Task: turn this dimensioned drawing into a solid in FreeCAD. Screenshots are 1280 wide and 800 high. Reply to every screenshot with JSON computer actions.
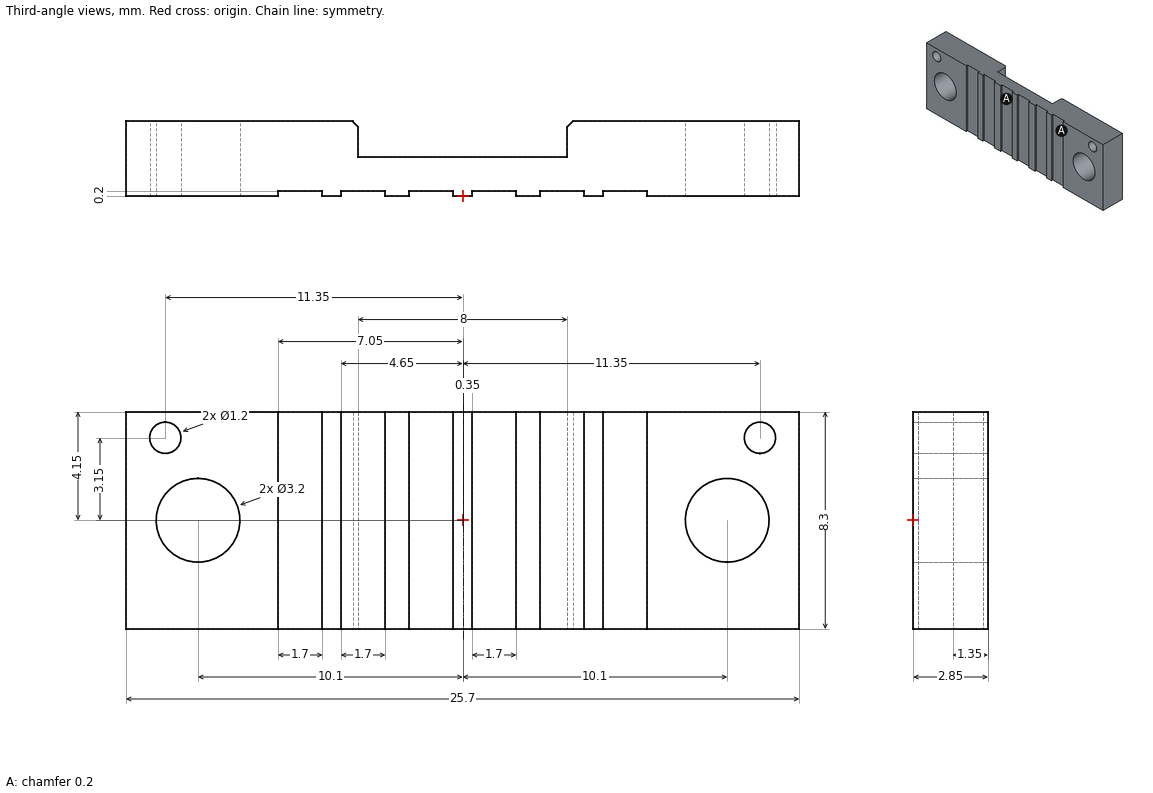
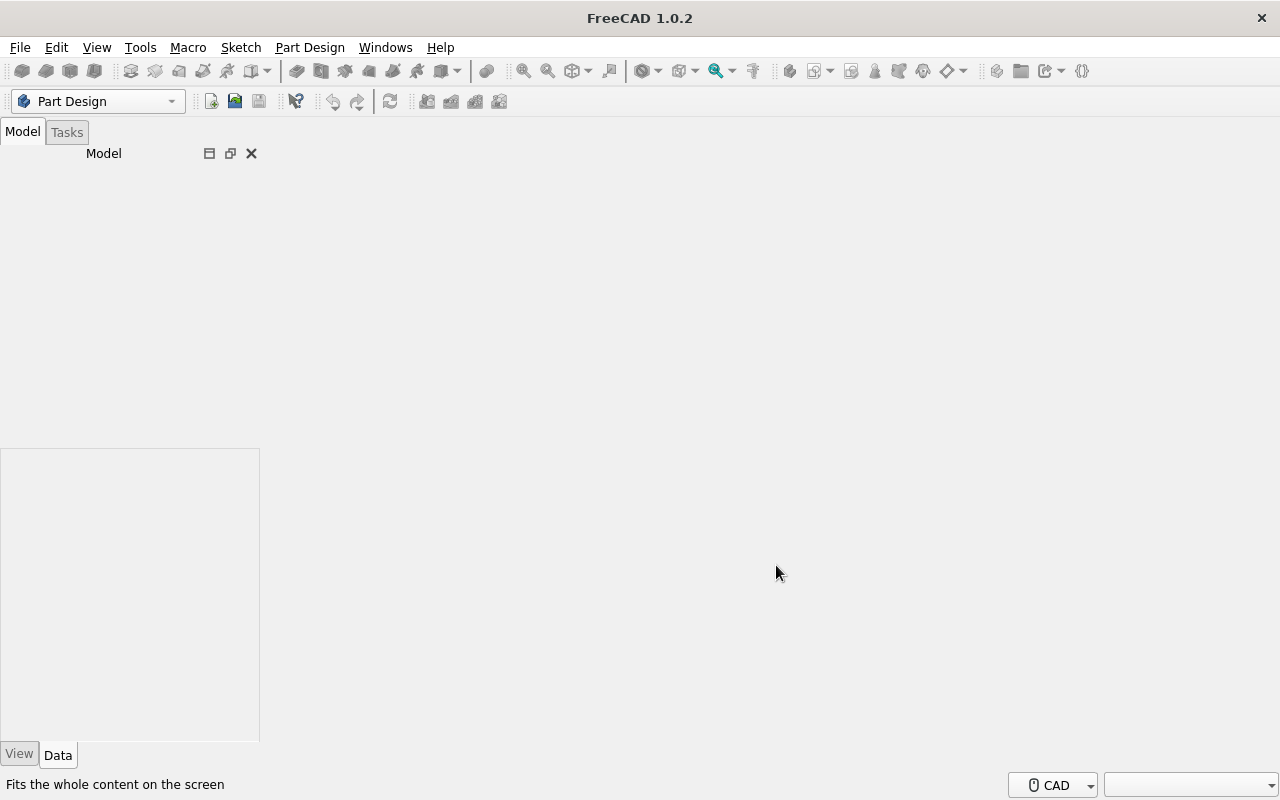
{"action": "left_click", "coordinate": [212, 102]}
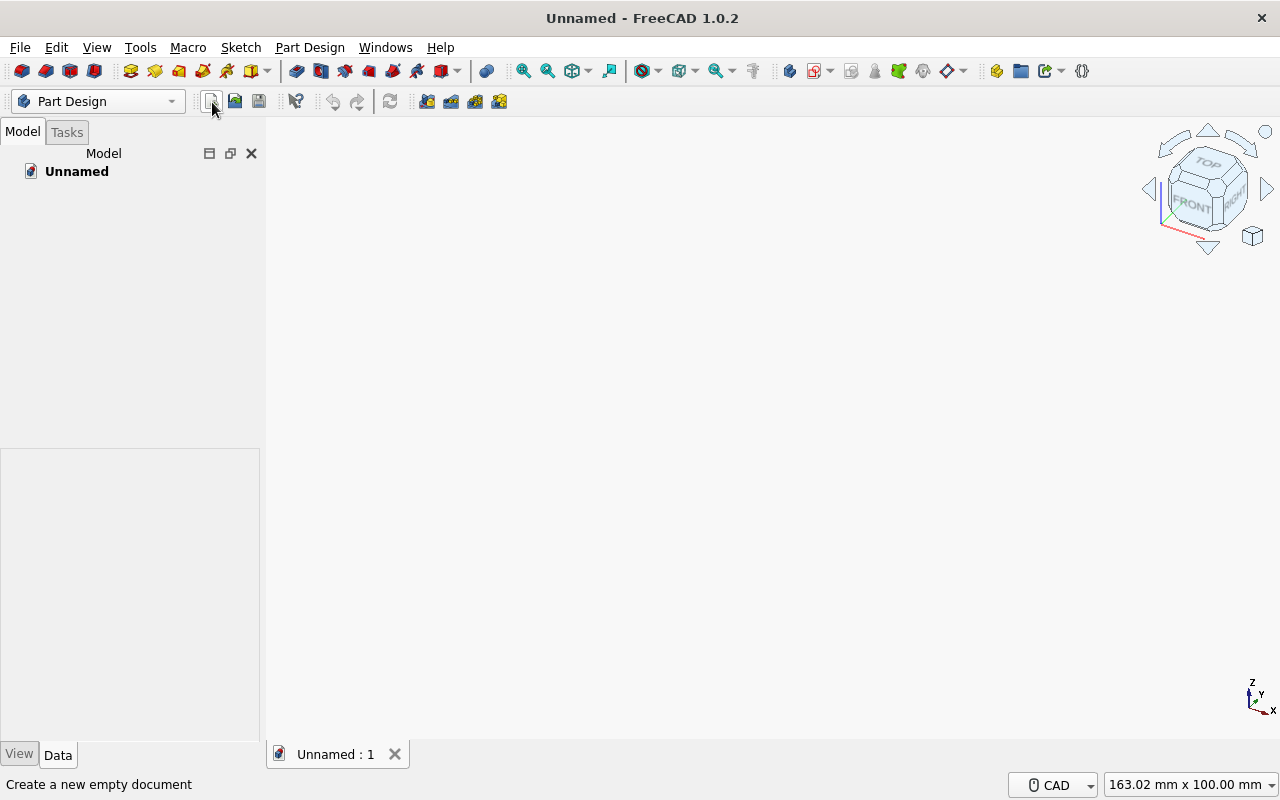
{"action": "left_click", "coordinate": [814, 72]}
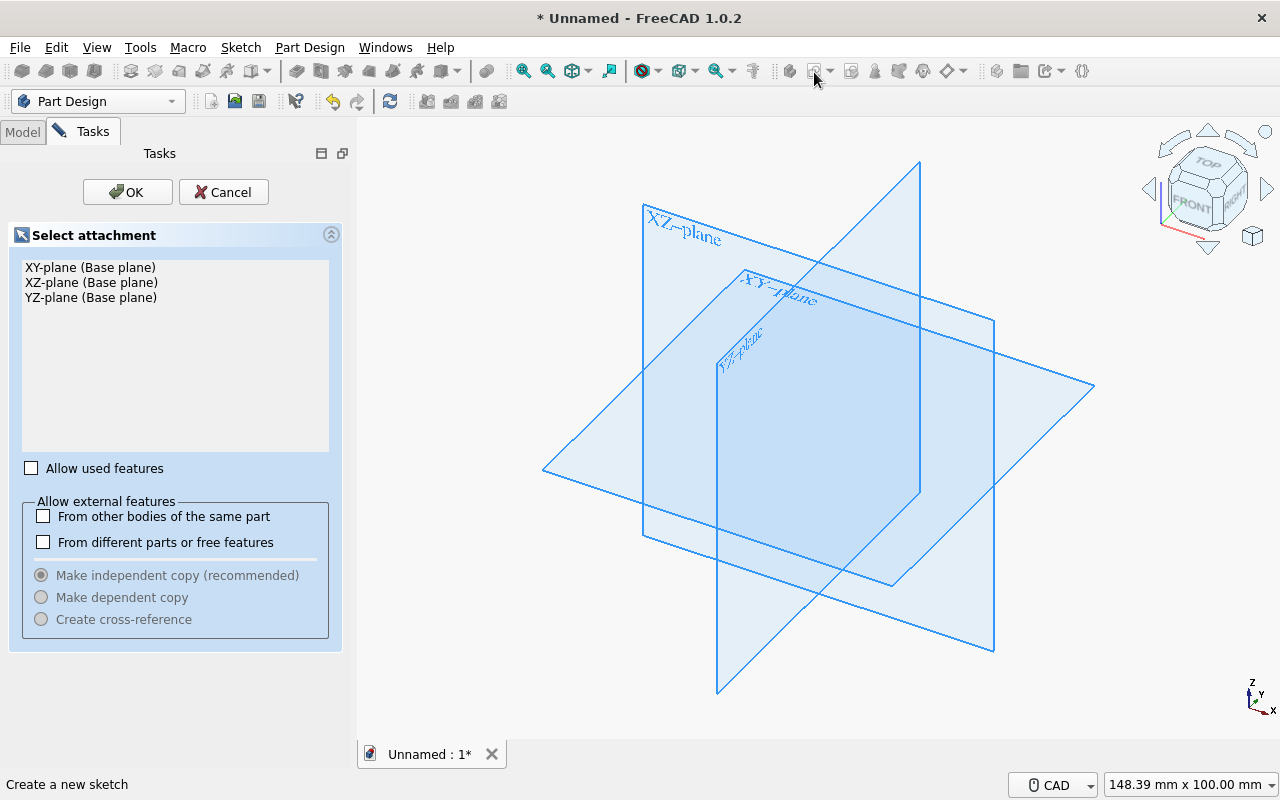
{"action": "left_click", "coordinate": [82, 282]}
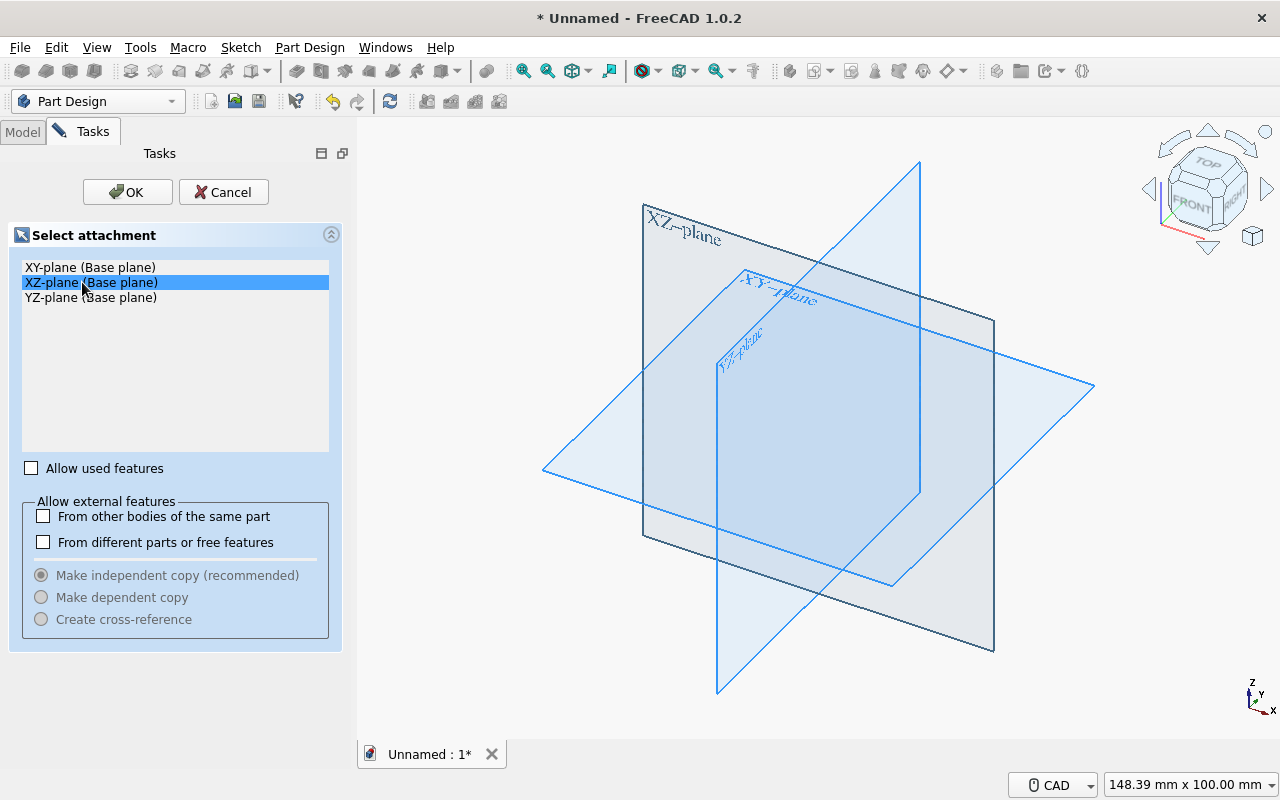
{"action": "left_click", "coordinate": [128, 192]}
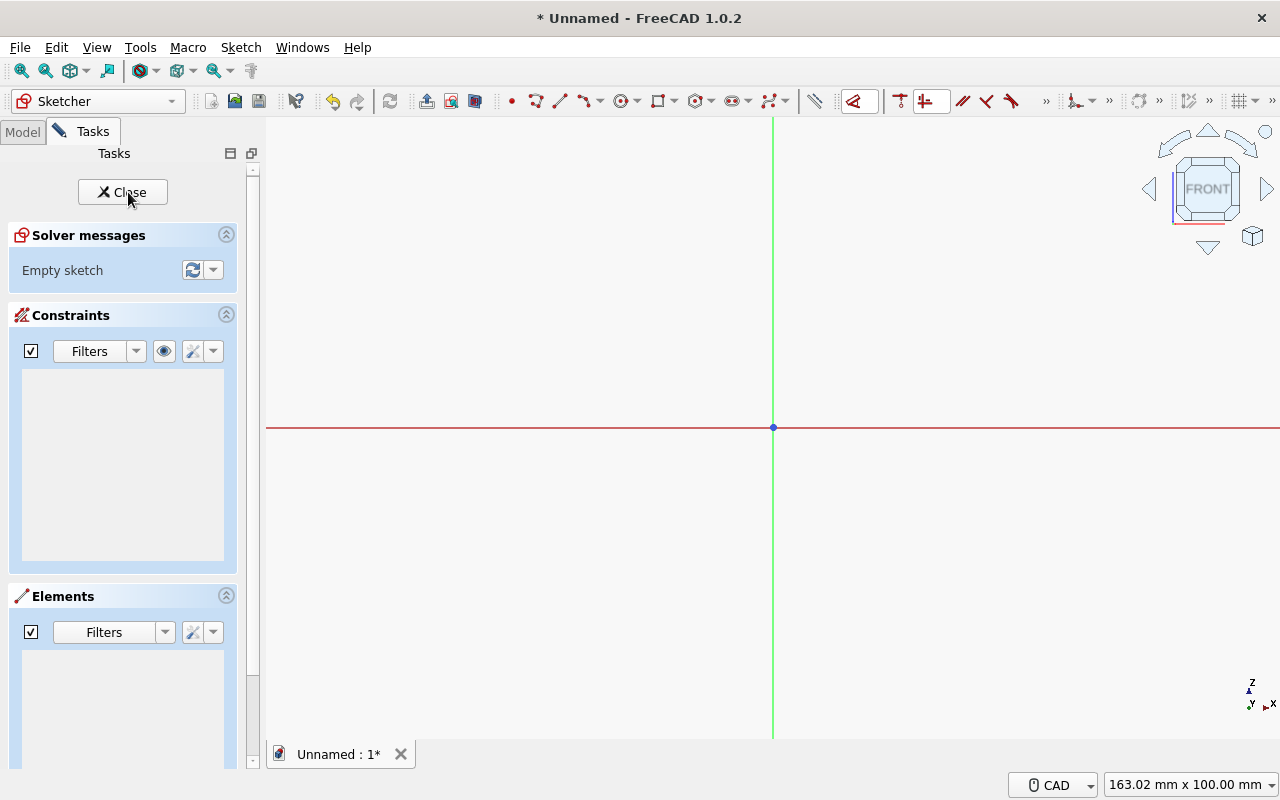
{"action": "scroll", "coordinate": [803, 428], "scroll_direction": "up", "scroll_amount": 6}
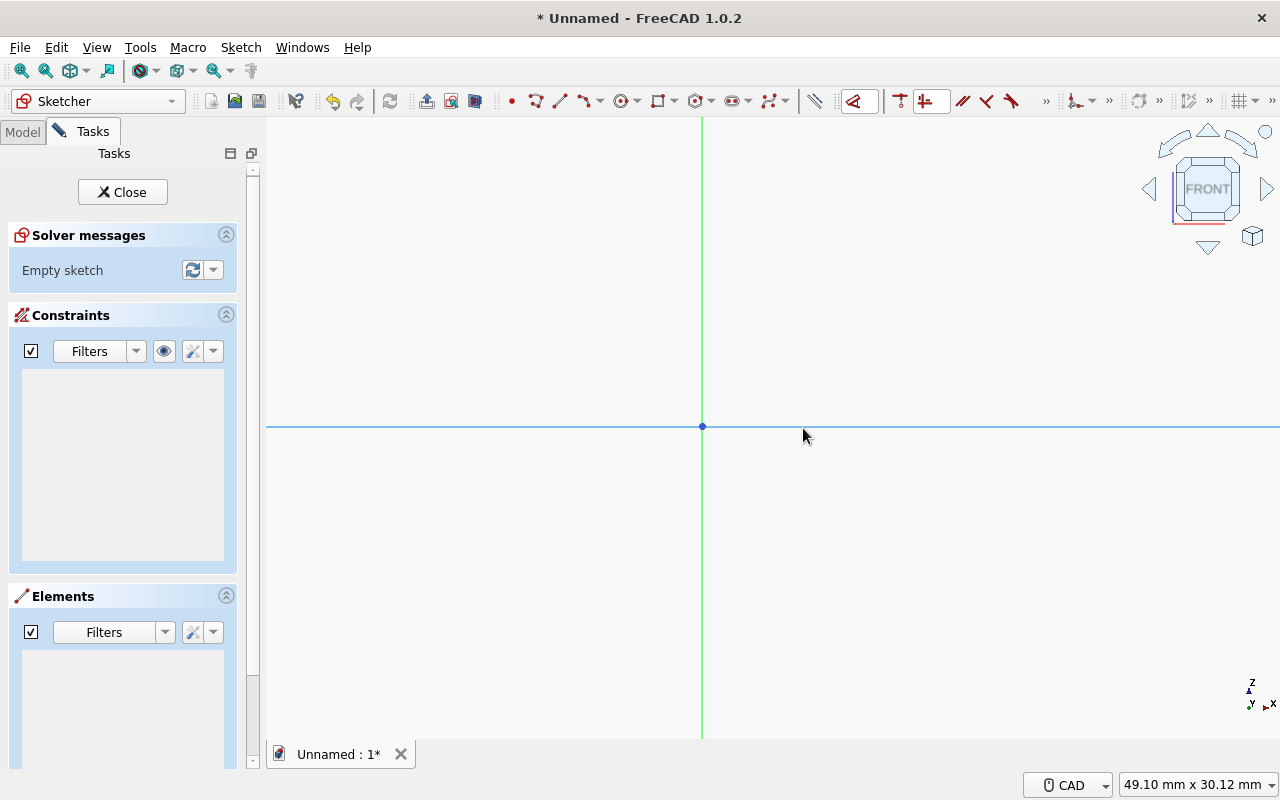
{"action": "key", "text": "g v"}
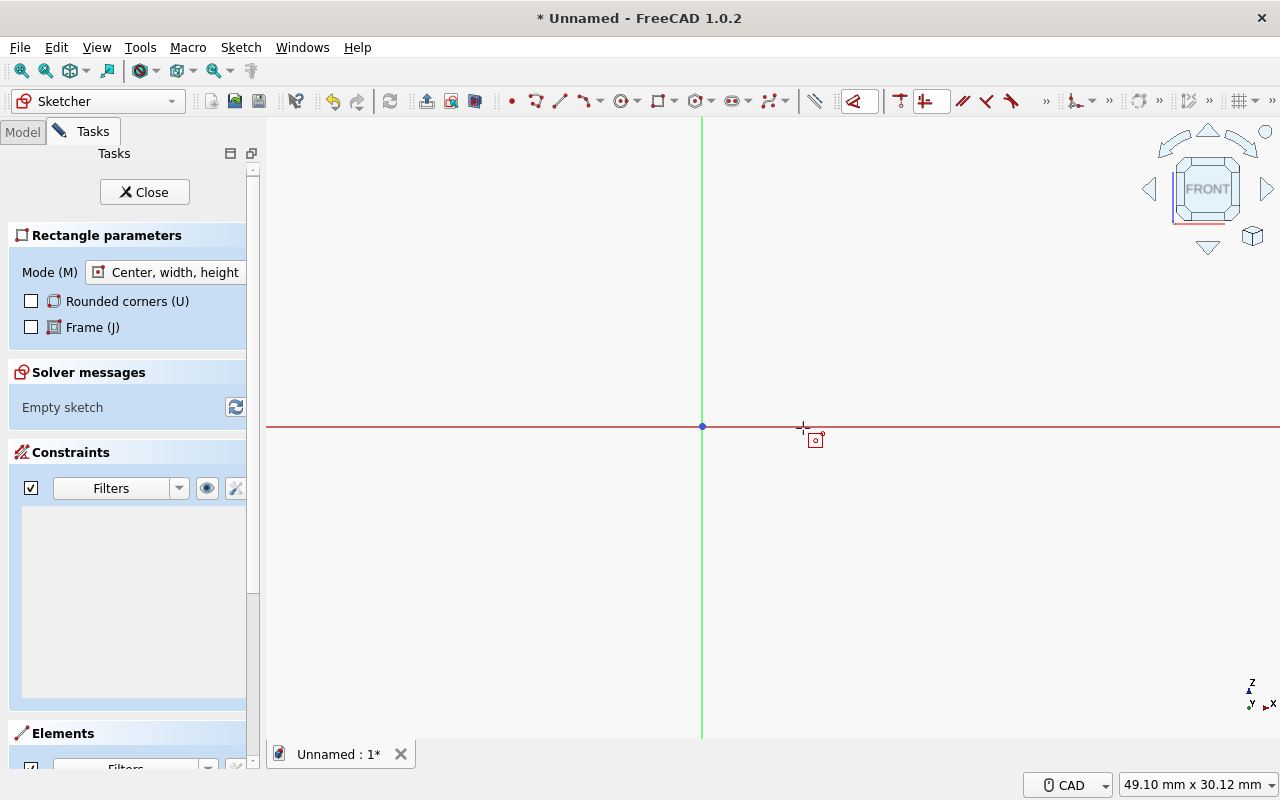
{"action": "left_click", "coordinate": [702, 427]}
{"action": "left_click", "coordinate": [968, 341]}
{"action": "key", "text": "Escape"}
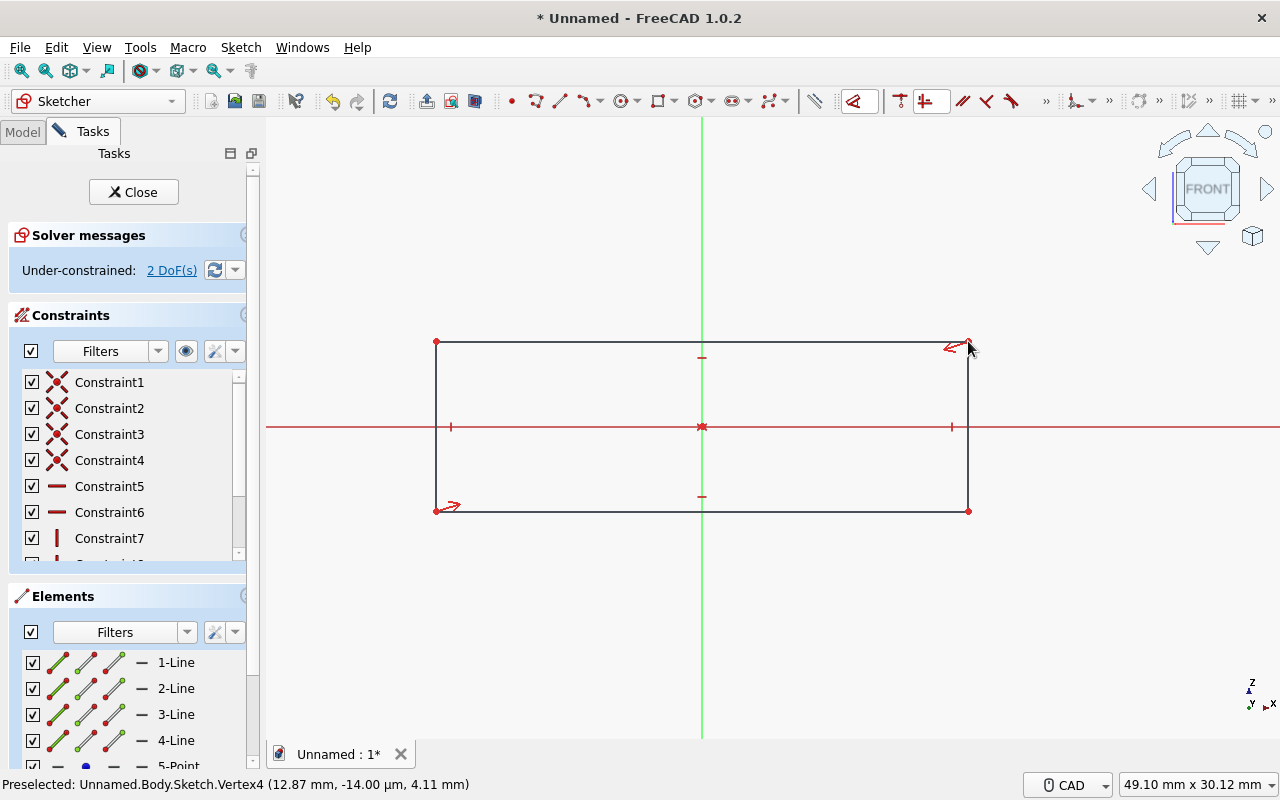
{"action": "key", "text": "d"}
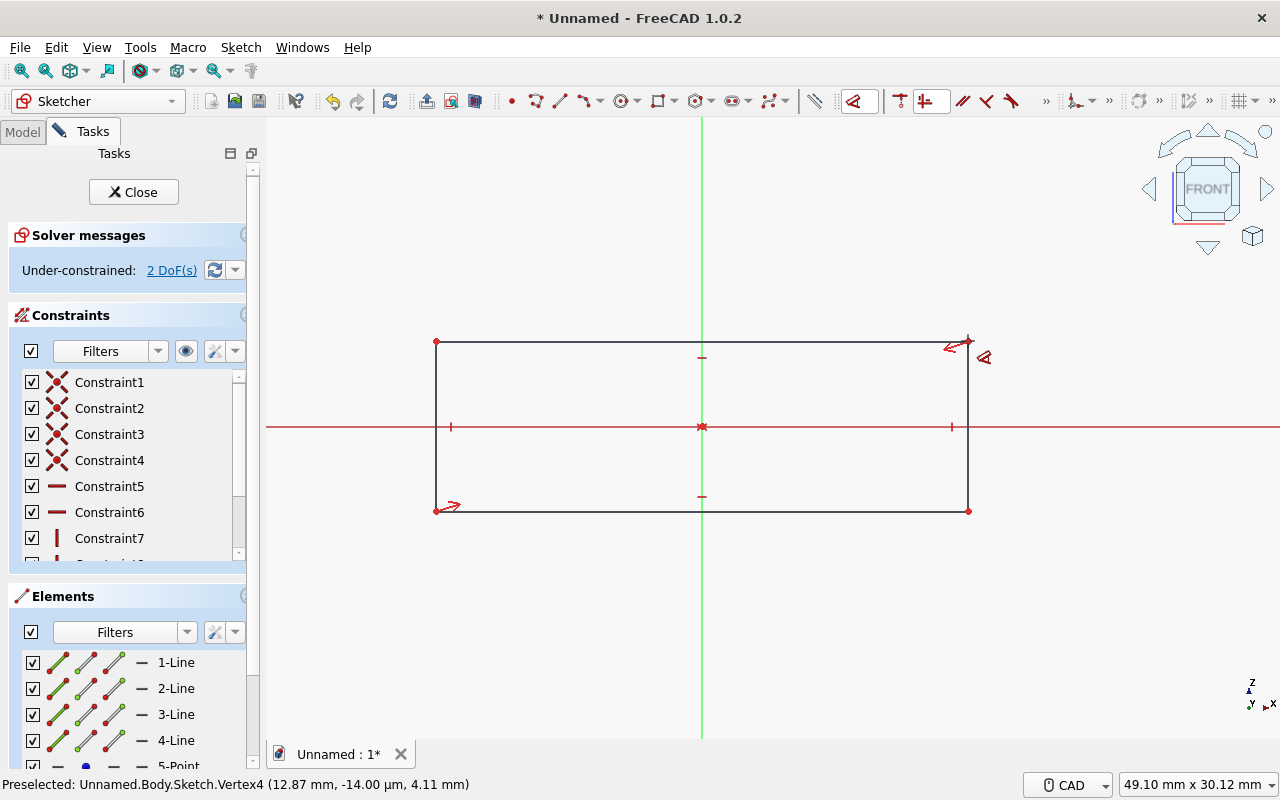
{"action": "left_click", "coordinate": [968, 461]}
{"action": "left_click", "coordinate": [1002, 388]}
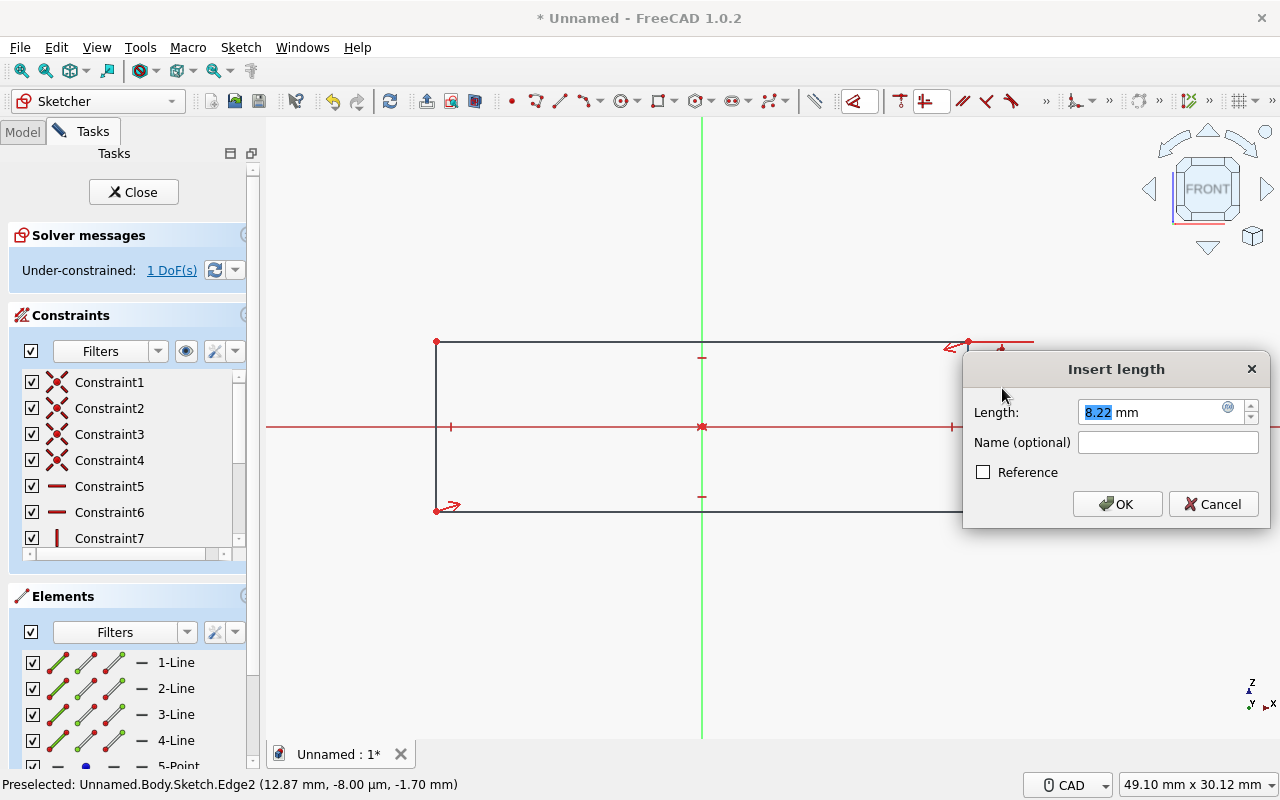
{"action": "type", "text": "8.3"}
{"action": "key", "text": "Return"}